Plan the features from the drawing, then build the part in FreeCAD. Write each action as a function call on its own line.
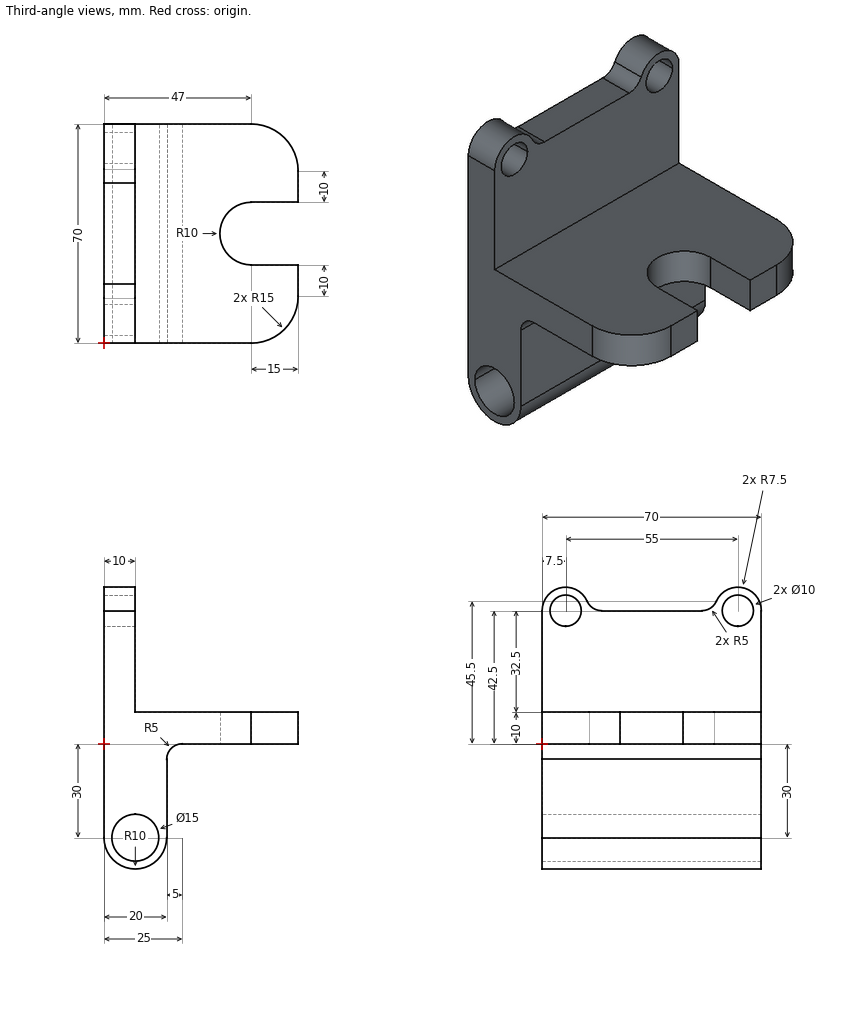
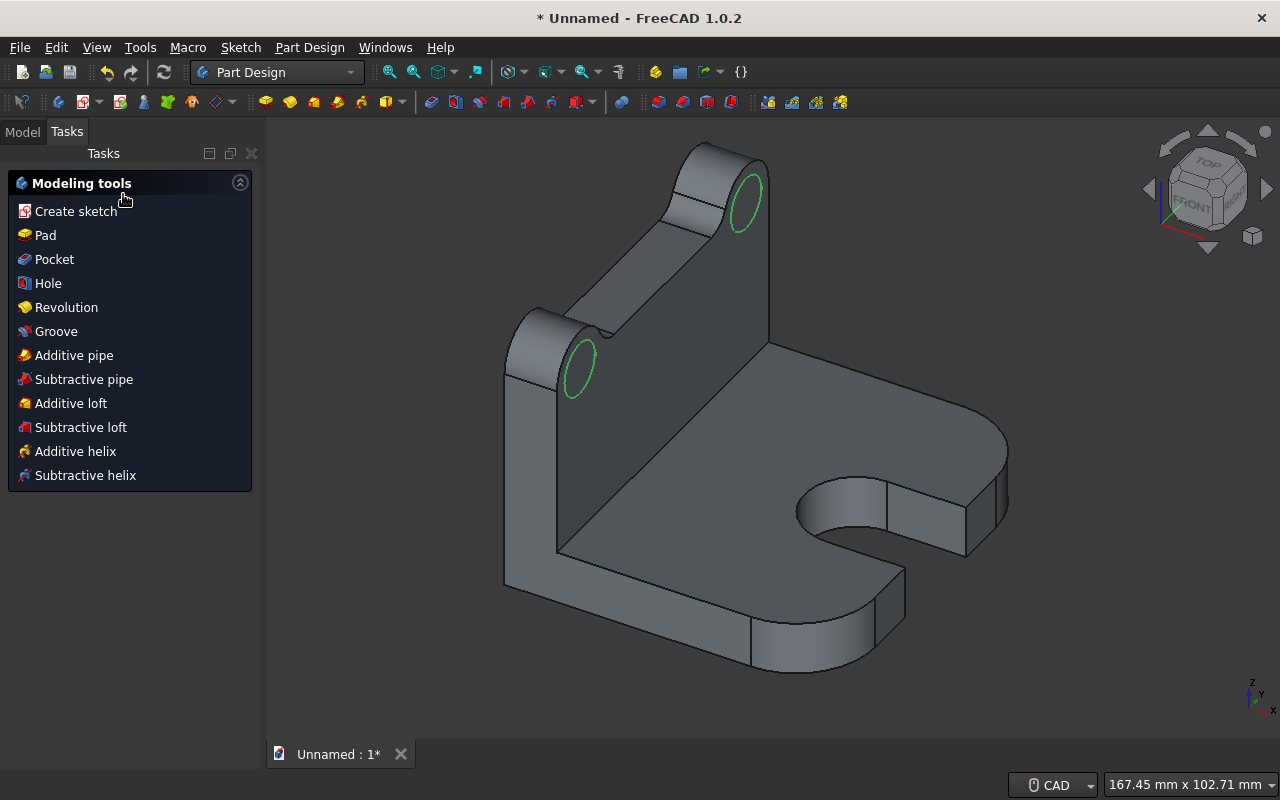
click(432, 102)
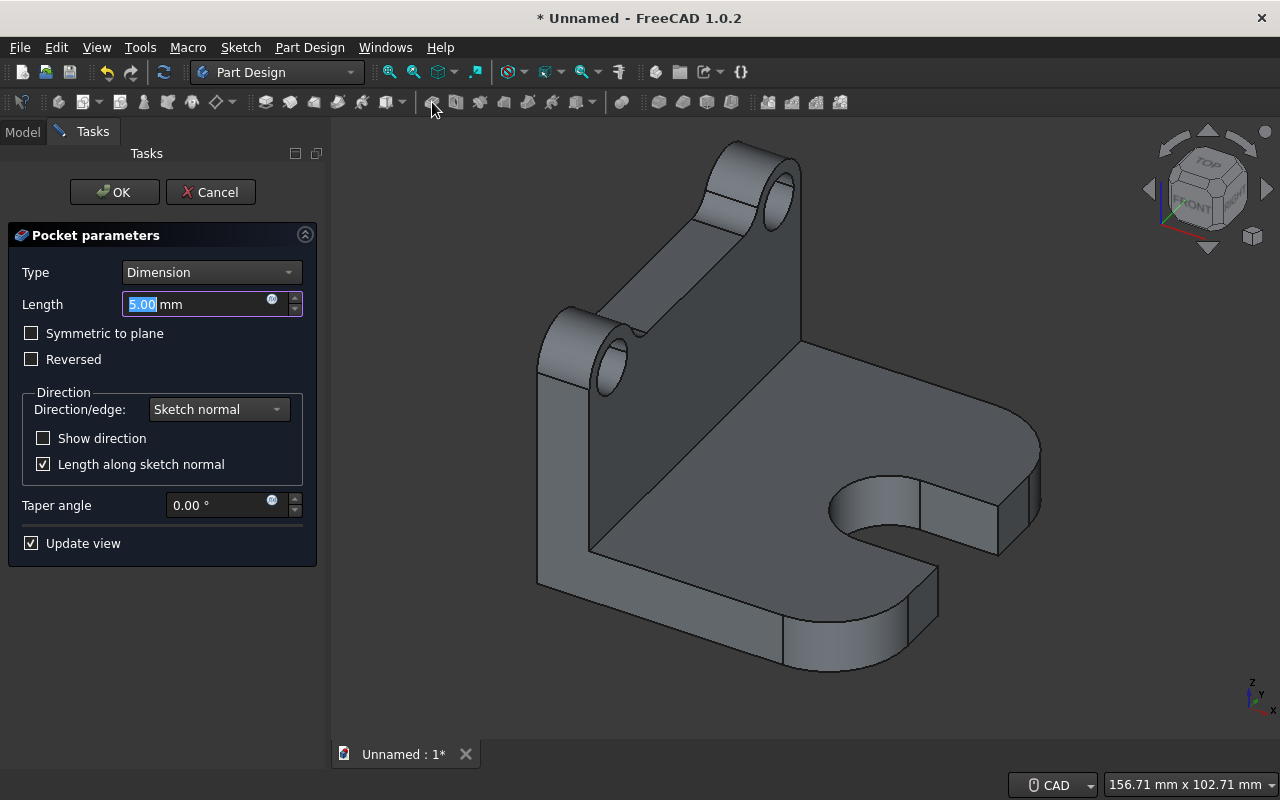
text(10)
key(Tab)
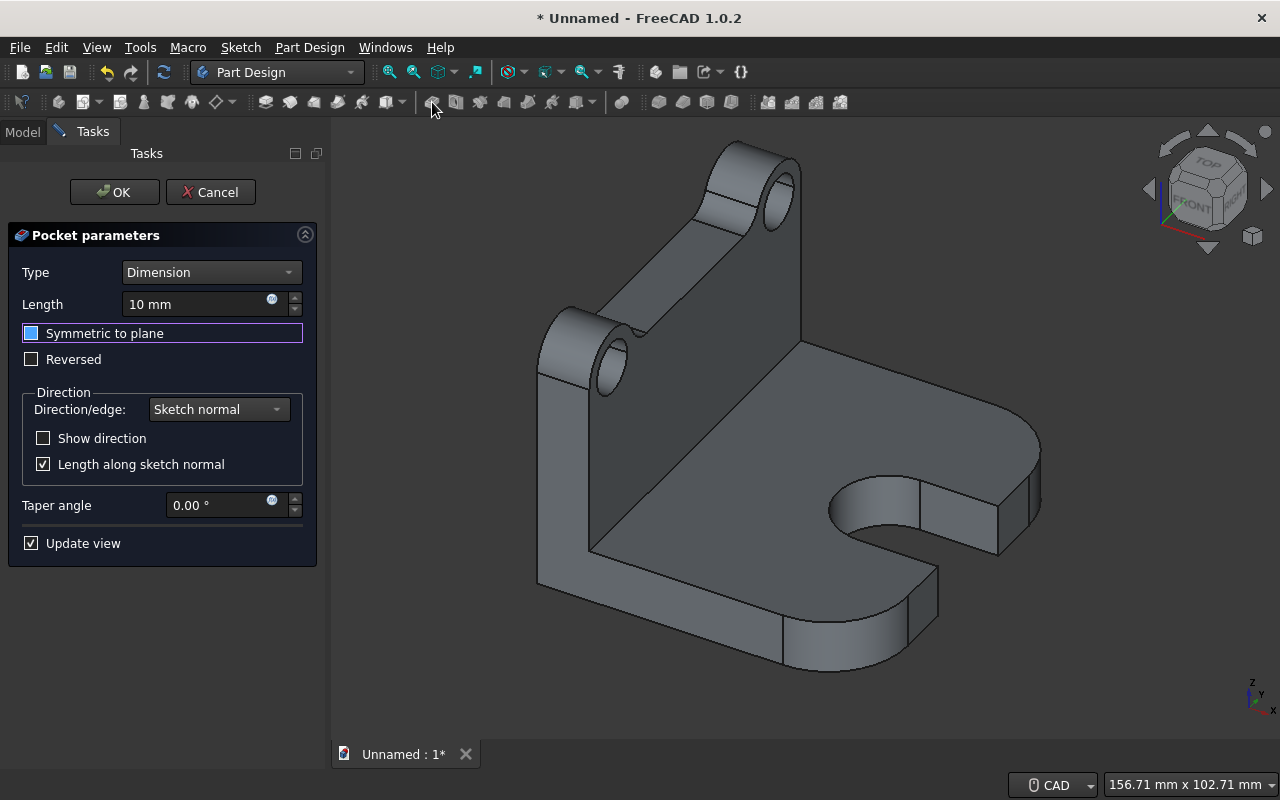
click(115, 192)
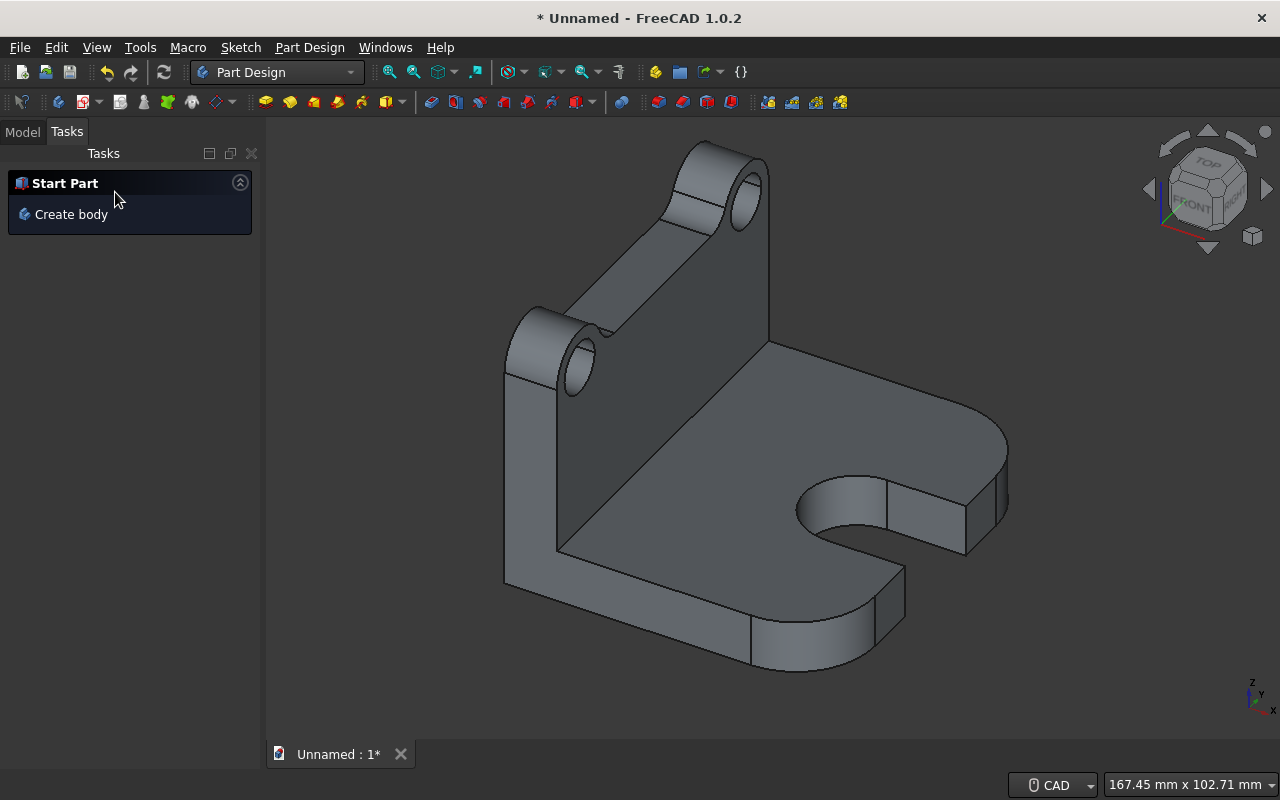
key(6)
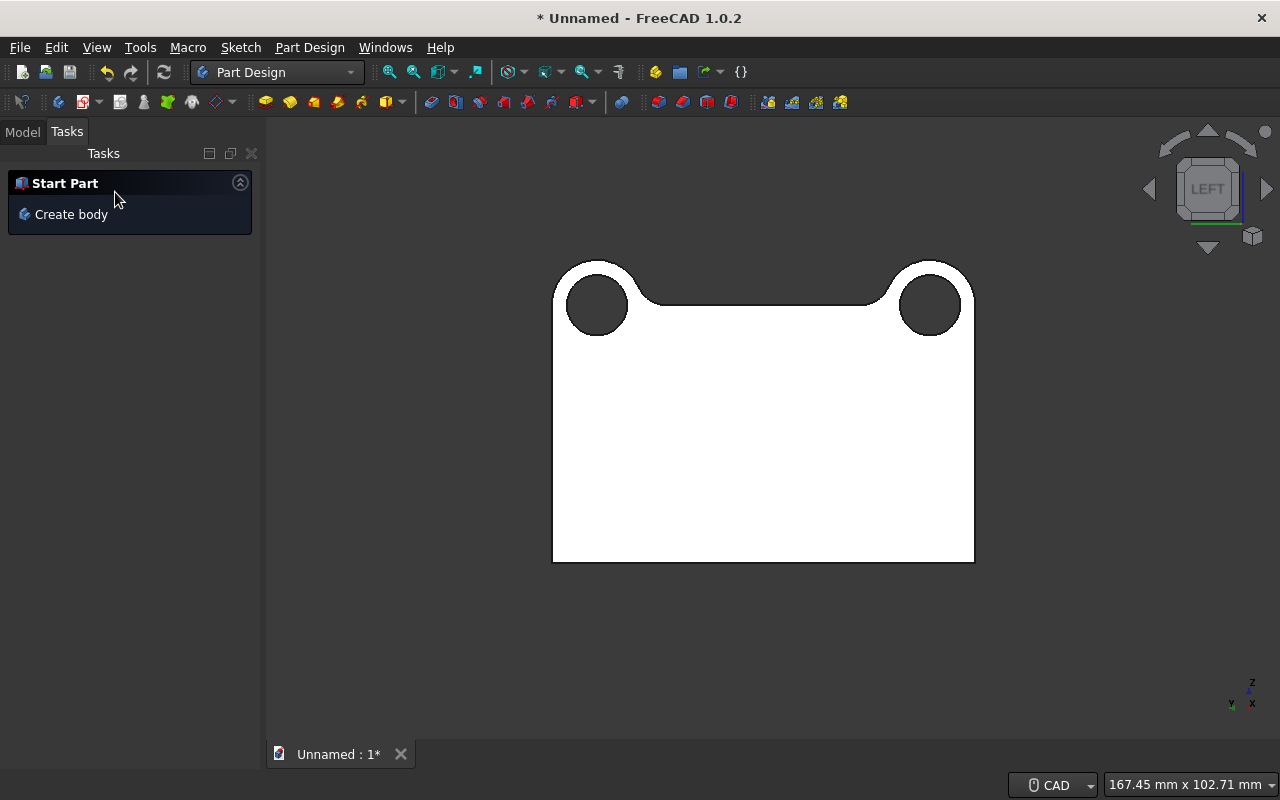
click(703, 453)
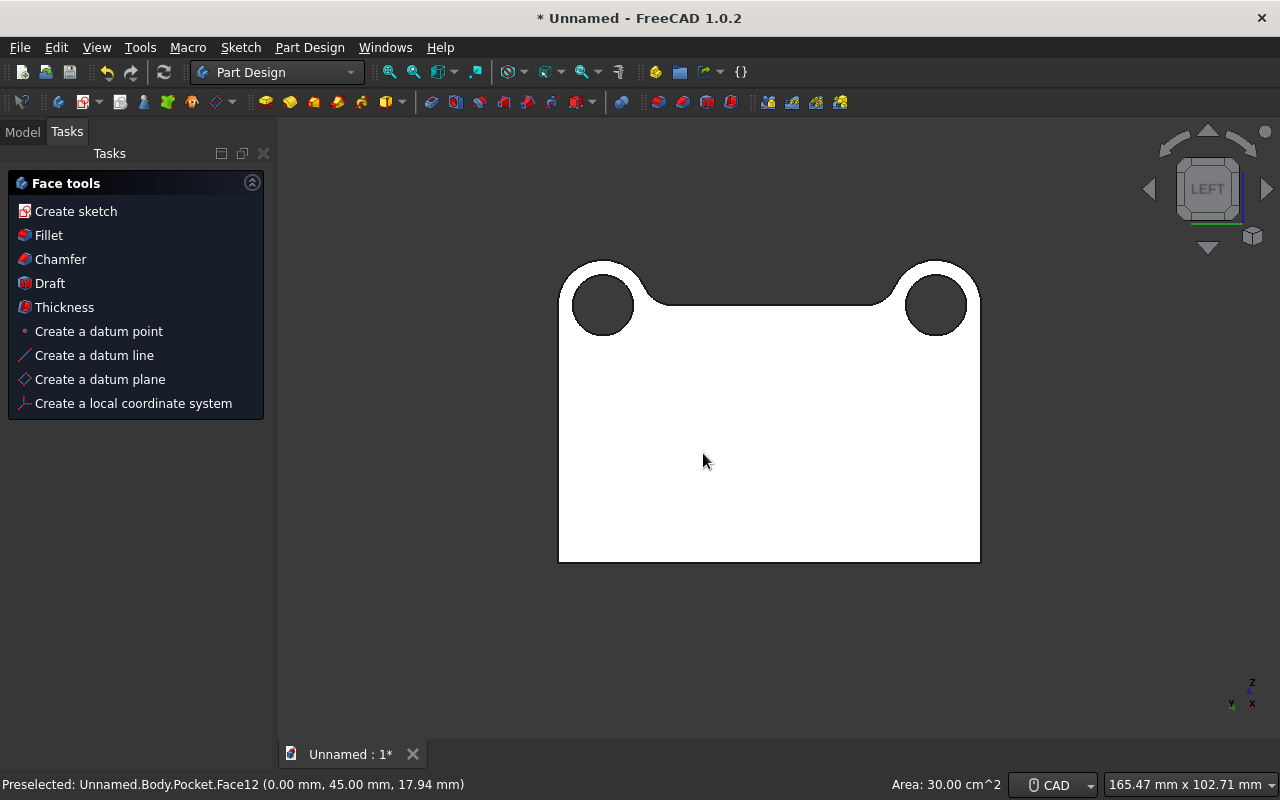
click(84, 102)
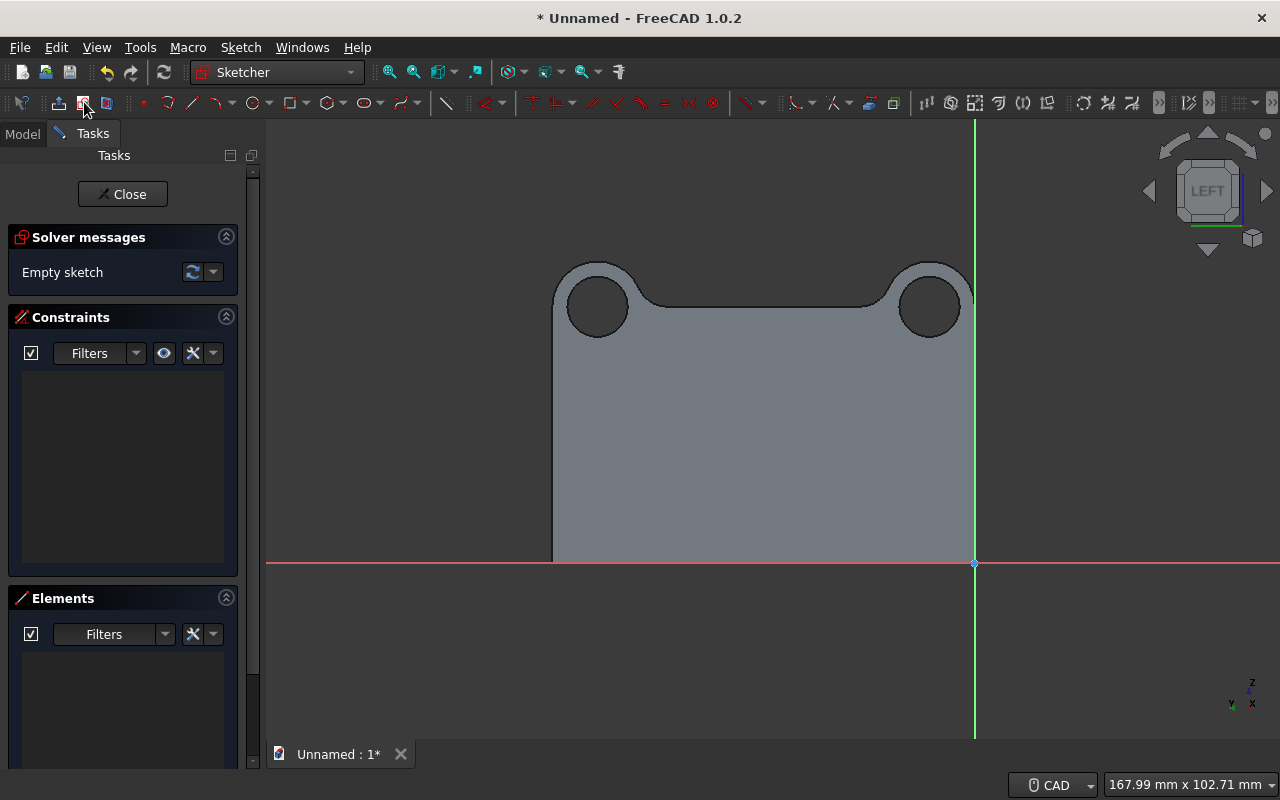
scroll(438, 147, down, 1)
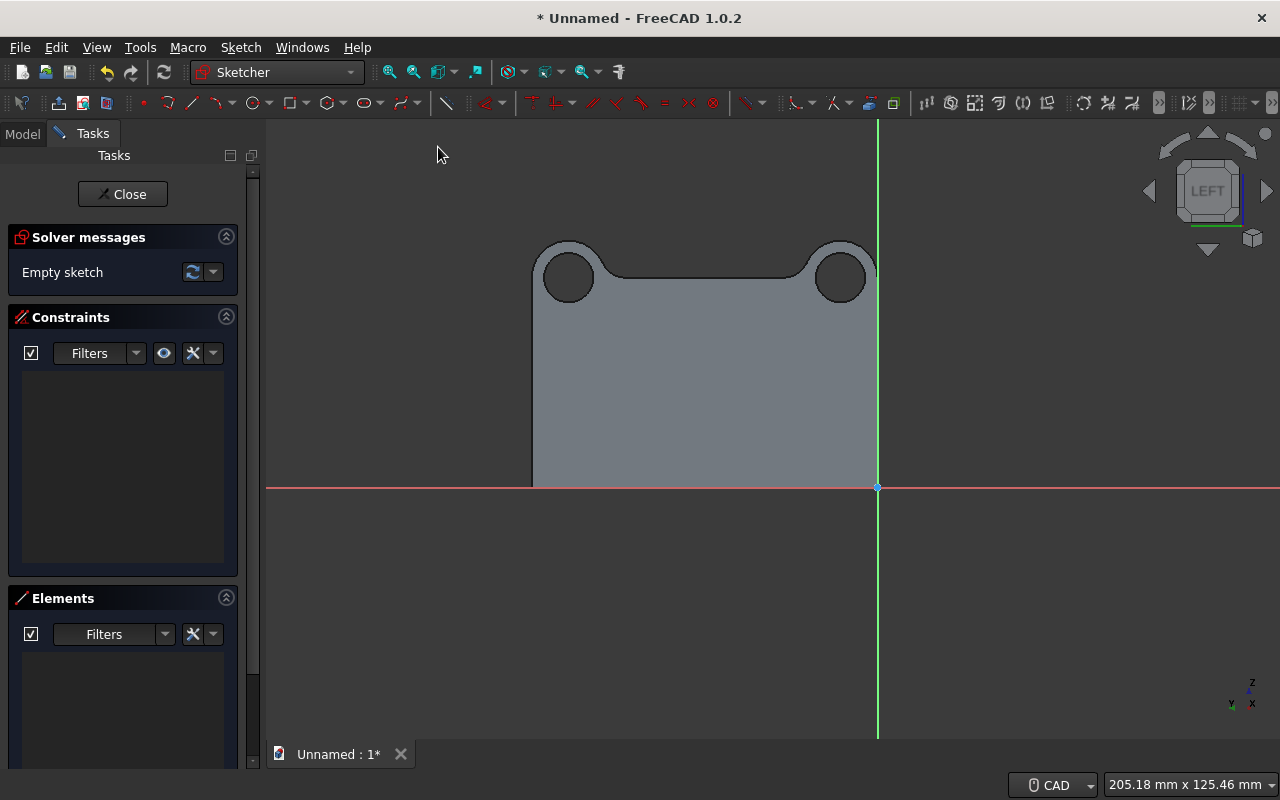
scroll(705, 711, up, 3)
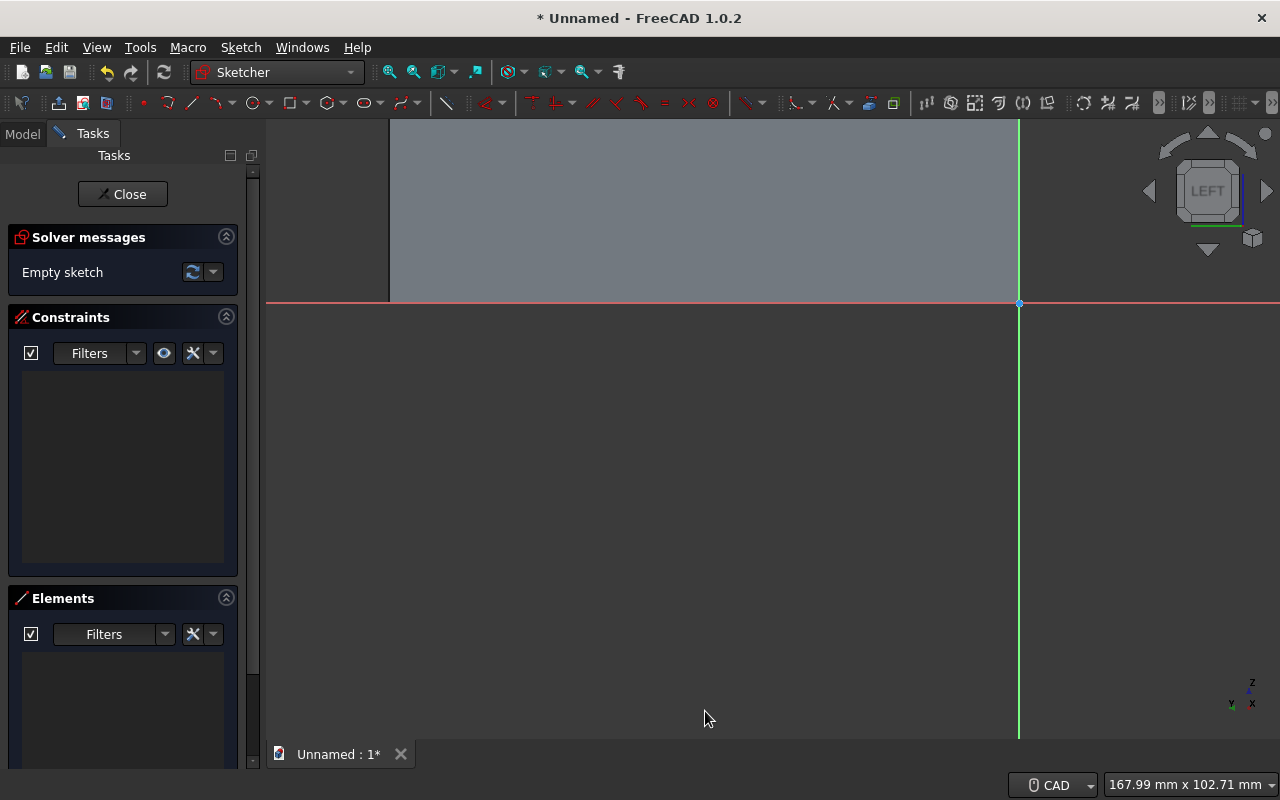
click(290, 104)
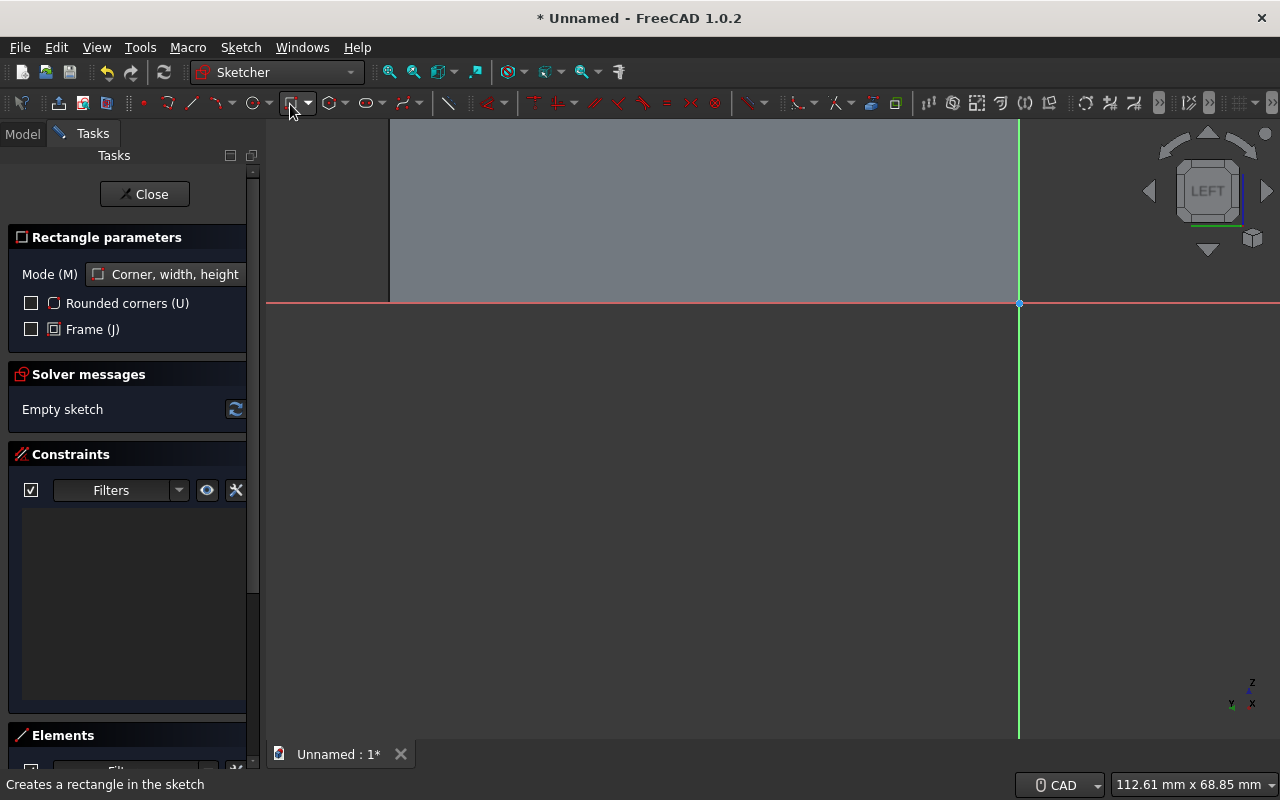
click(1019, 303)
click(389, 574)
key(Escape)